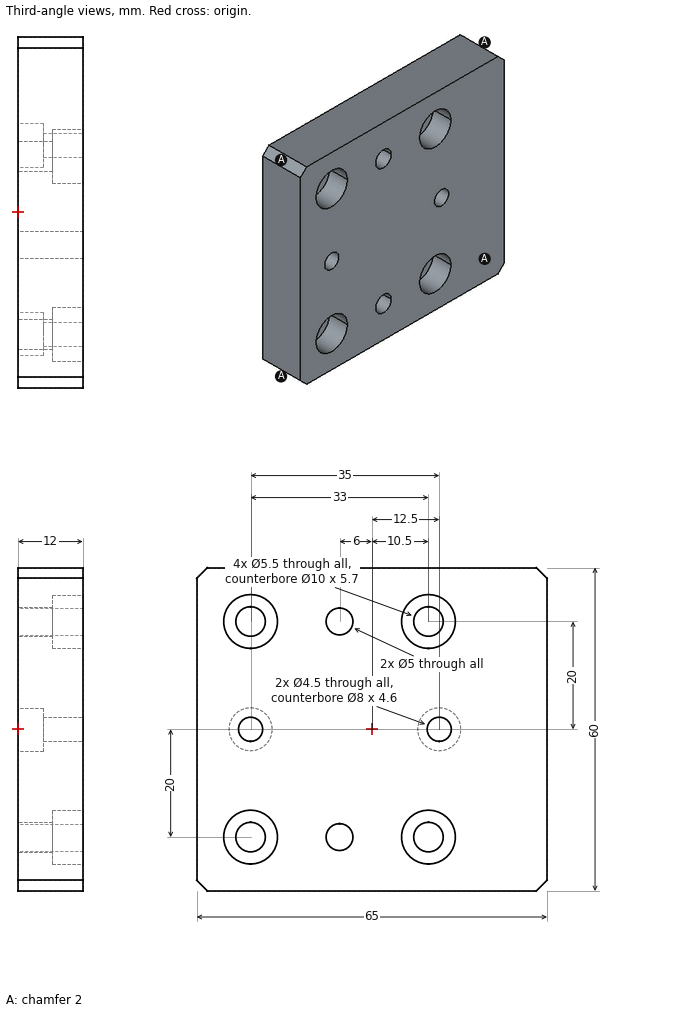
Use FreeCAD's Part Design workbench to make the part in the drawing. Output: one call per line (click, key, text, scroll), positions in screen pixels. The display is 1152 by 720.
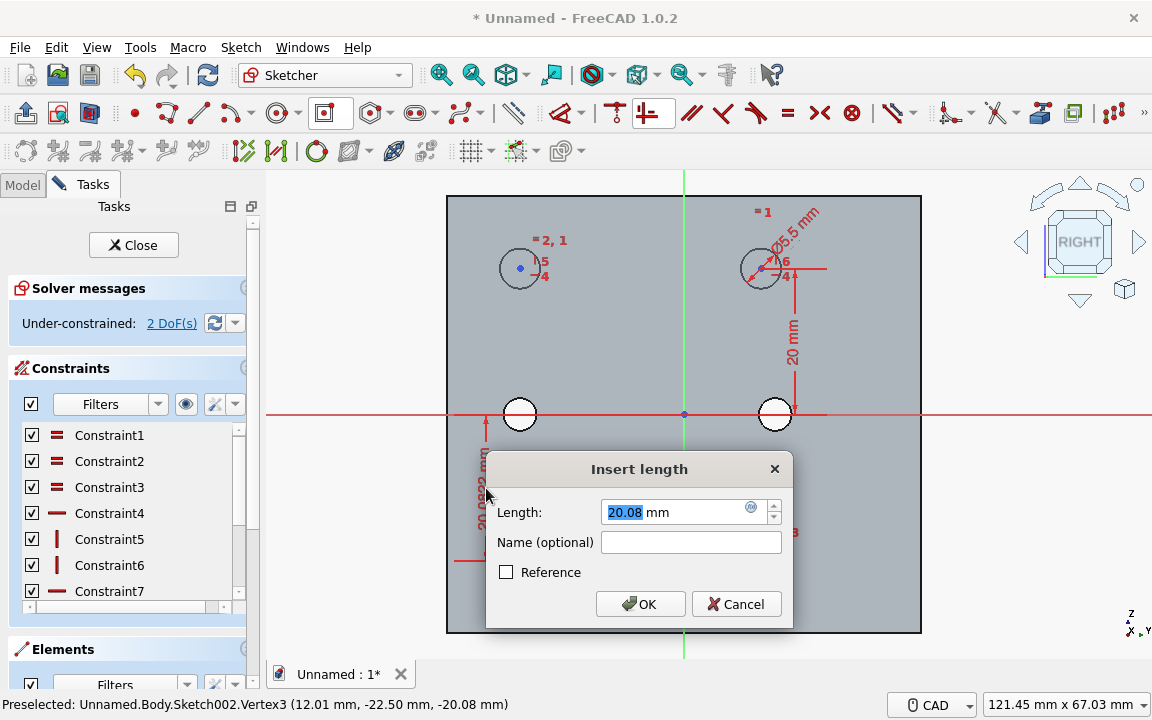
text(20)
key(Return)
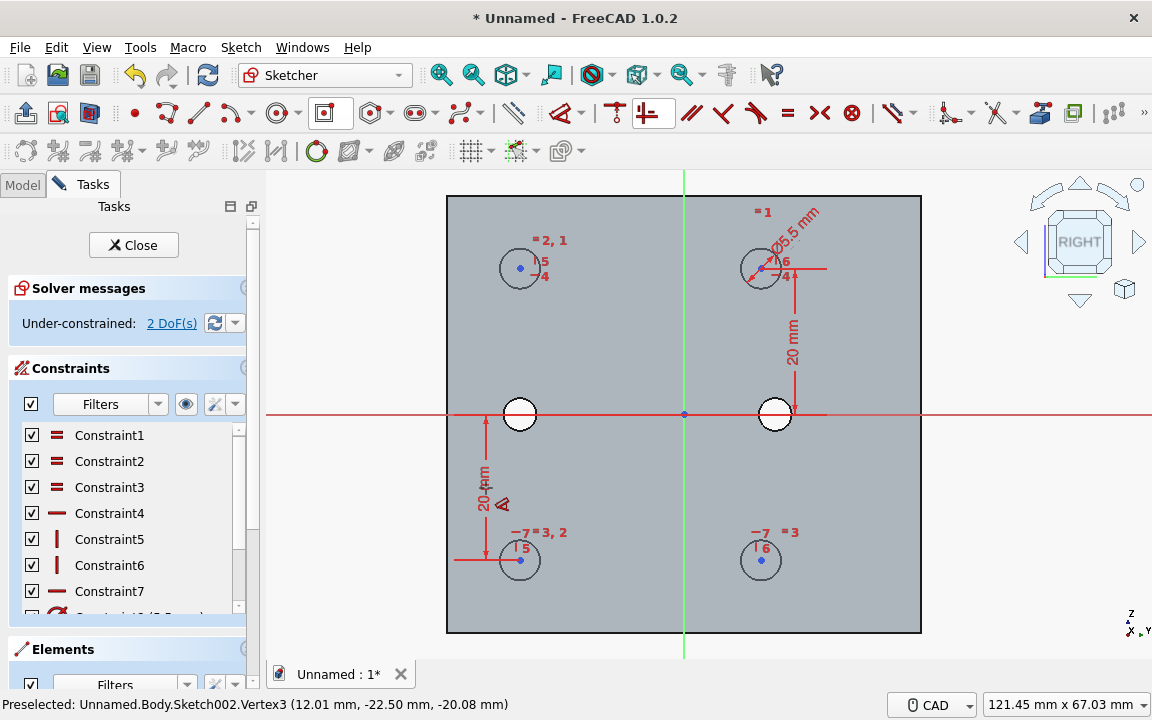
click(761, 269)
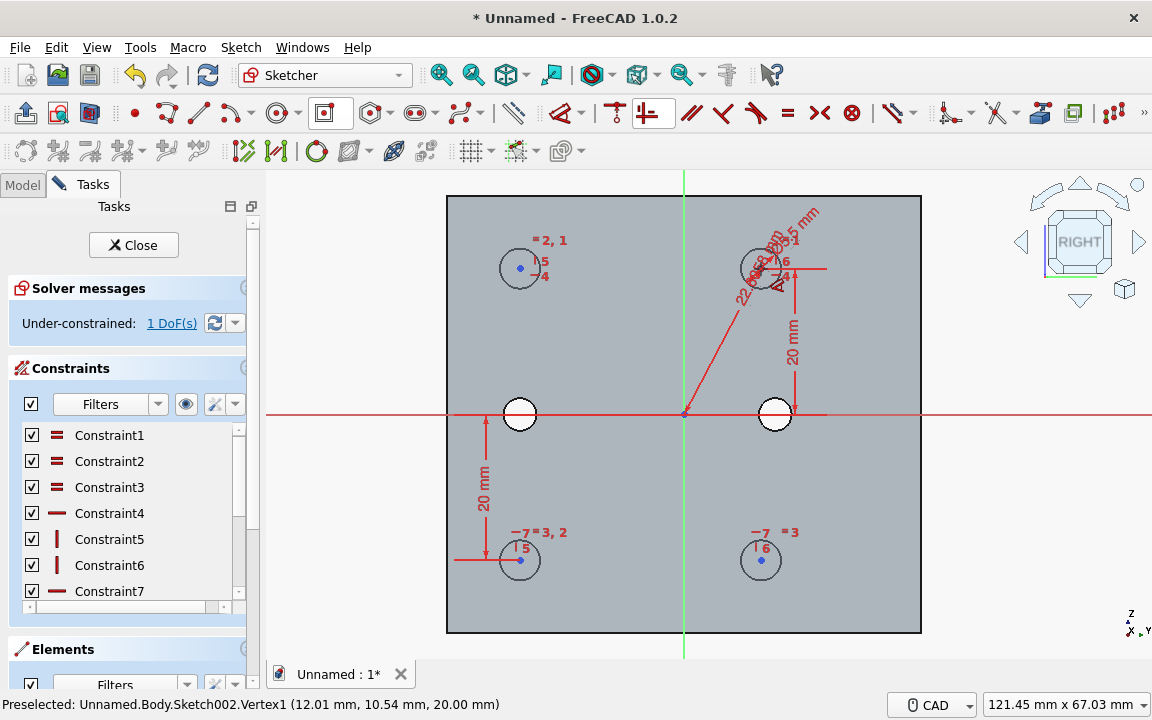
click(520, 269)
click(641, 235)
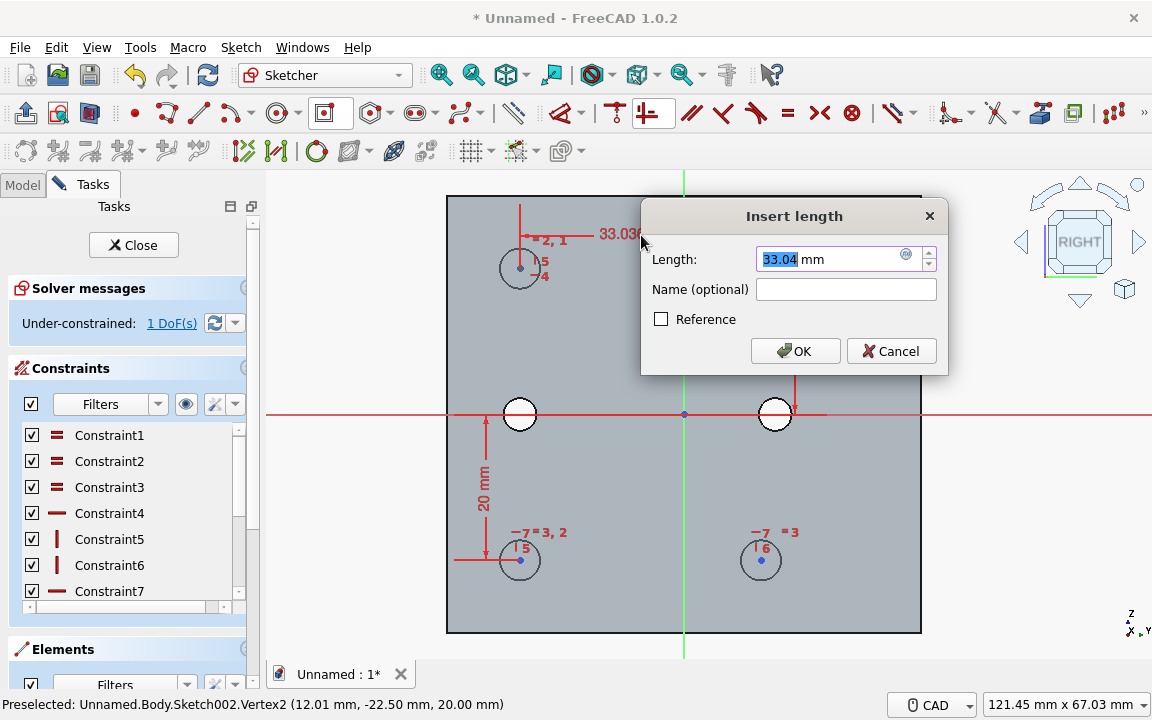
text(33)
key(Return)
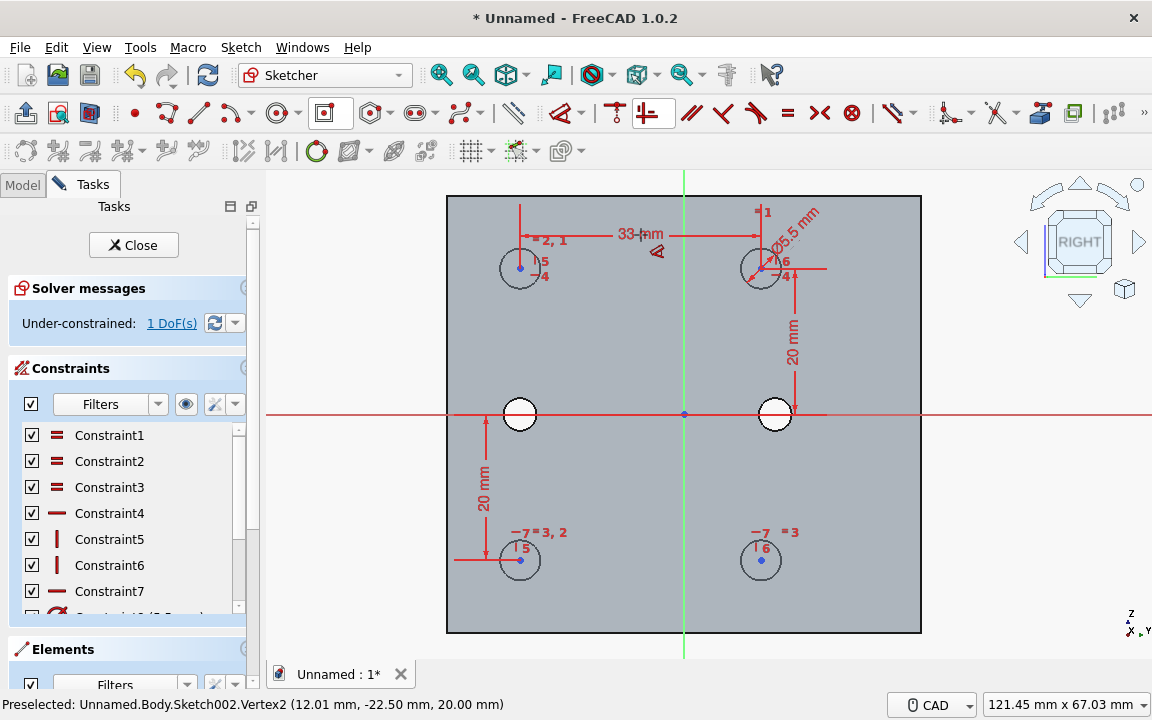
click(761, 269)
click(723, 235)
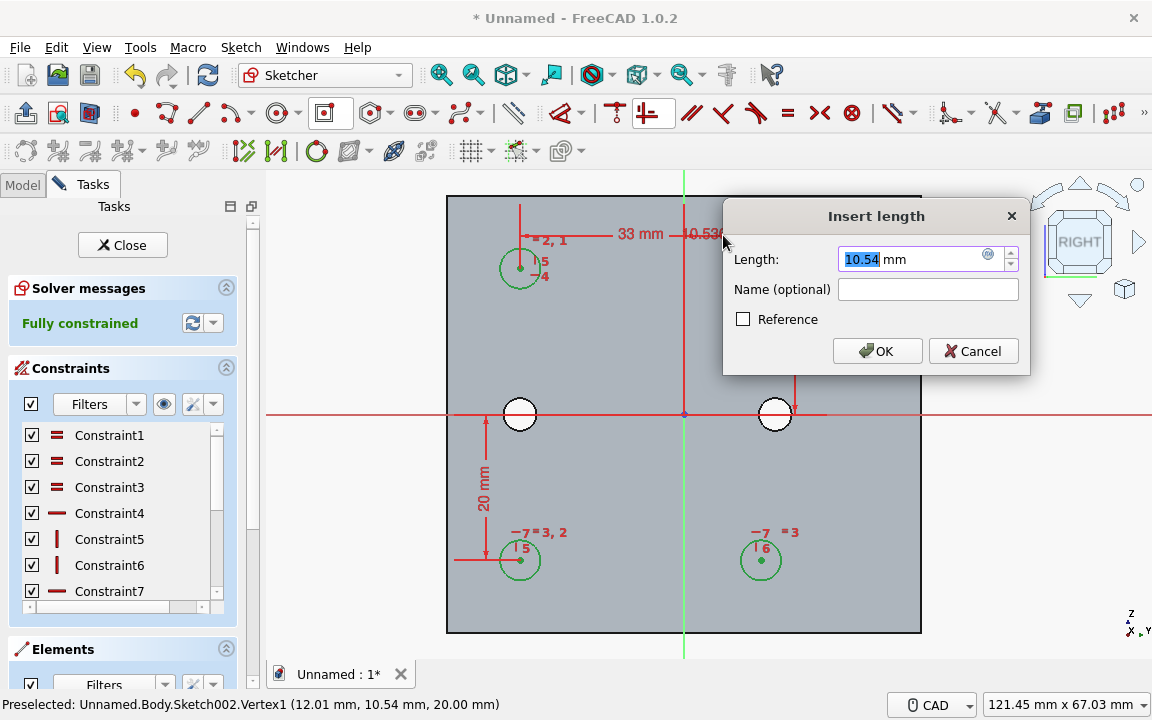
text(10.5)
key(Return)
key(Escape)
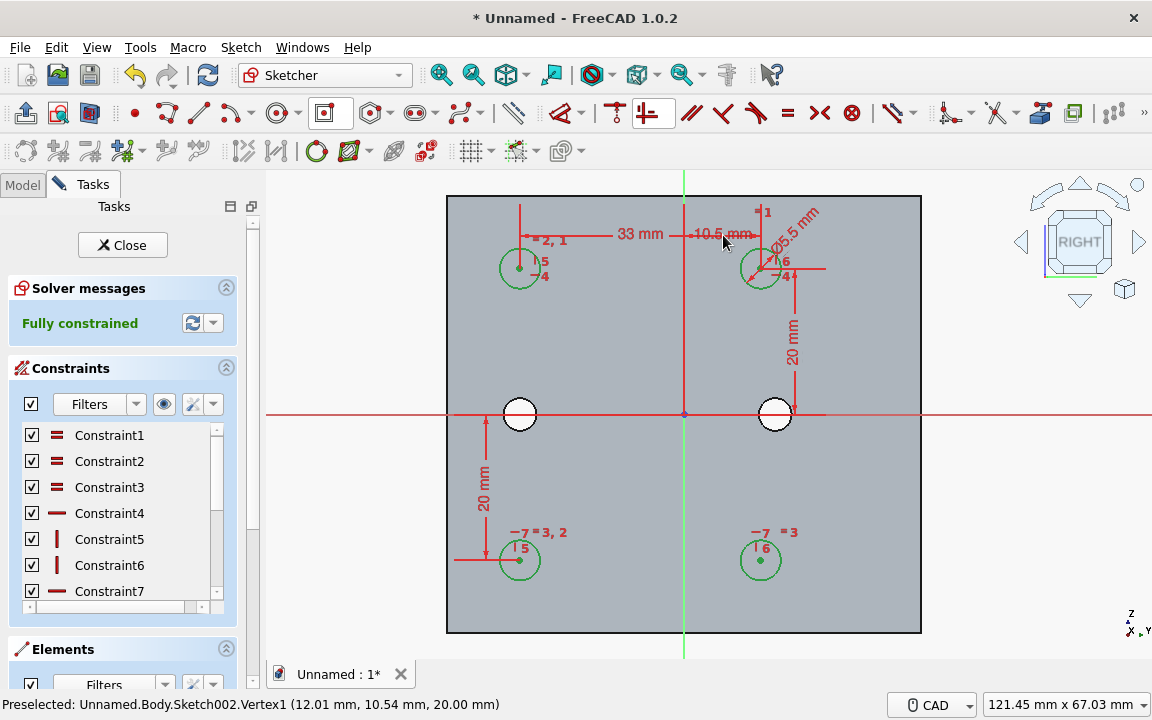
click(123, 245)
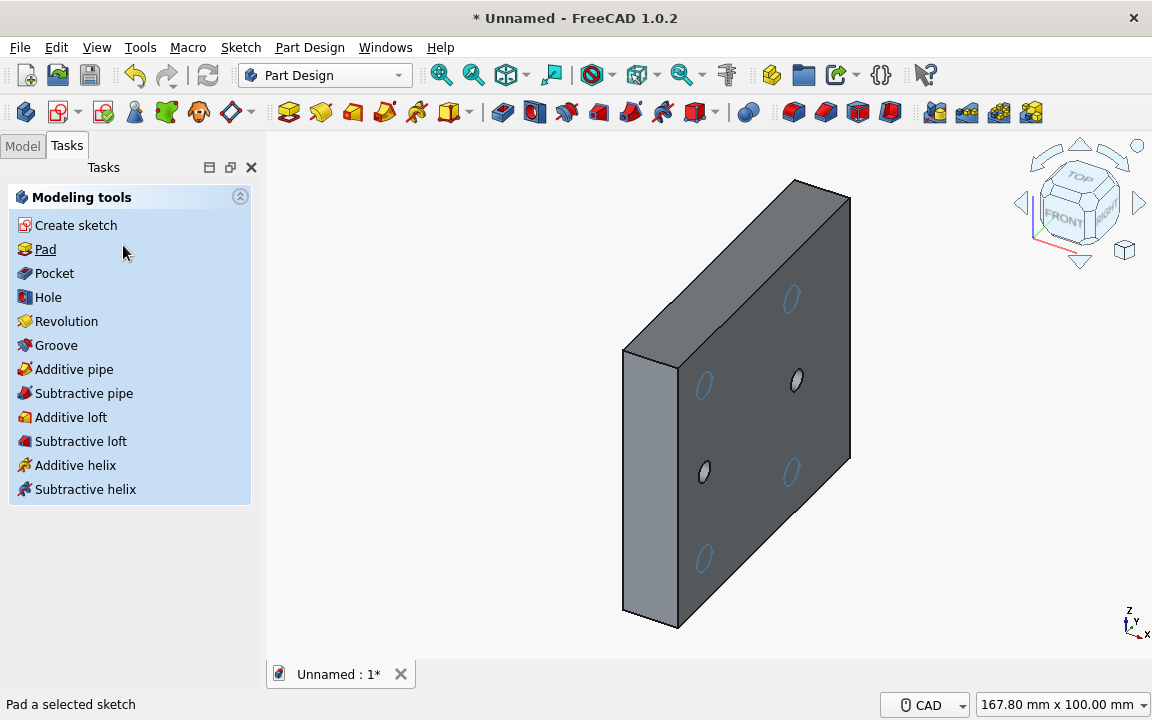
click(536, 112)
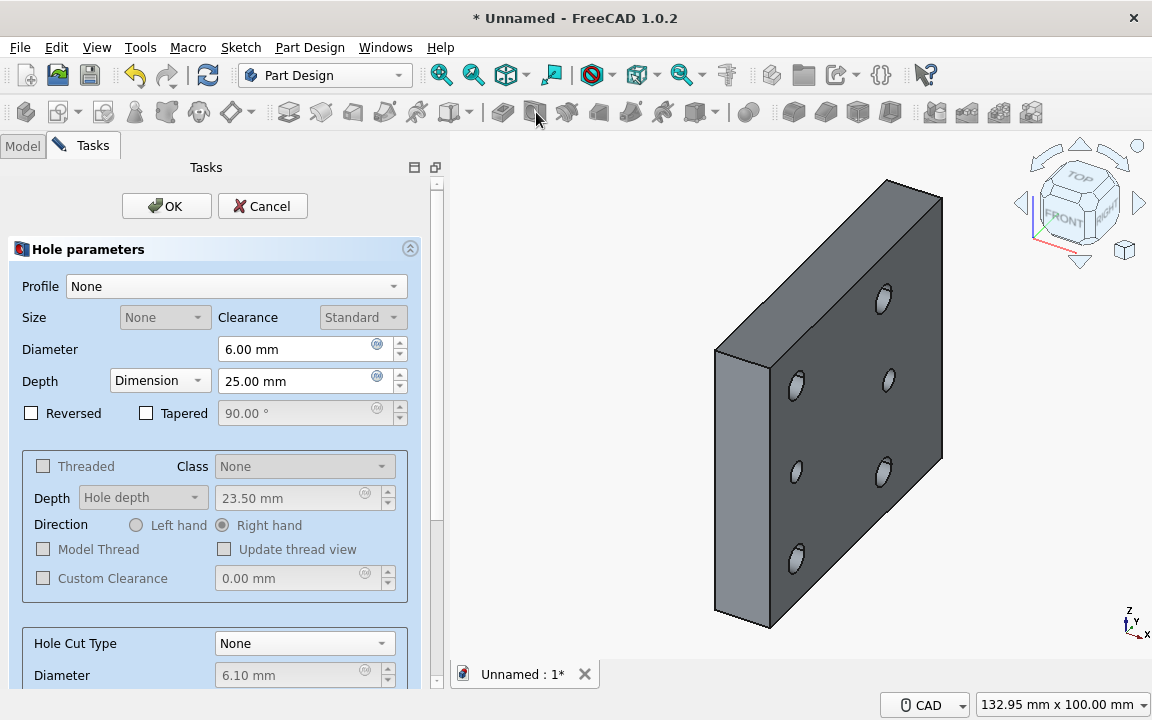
triple_click(305, 349)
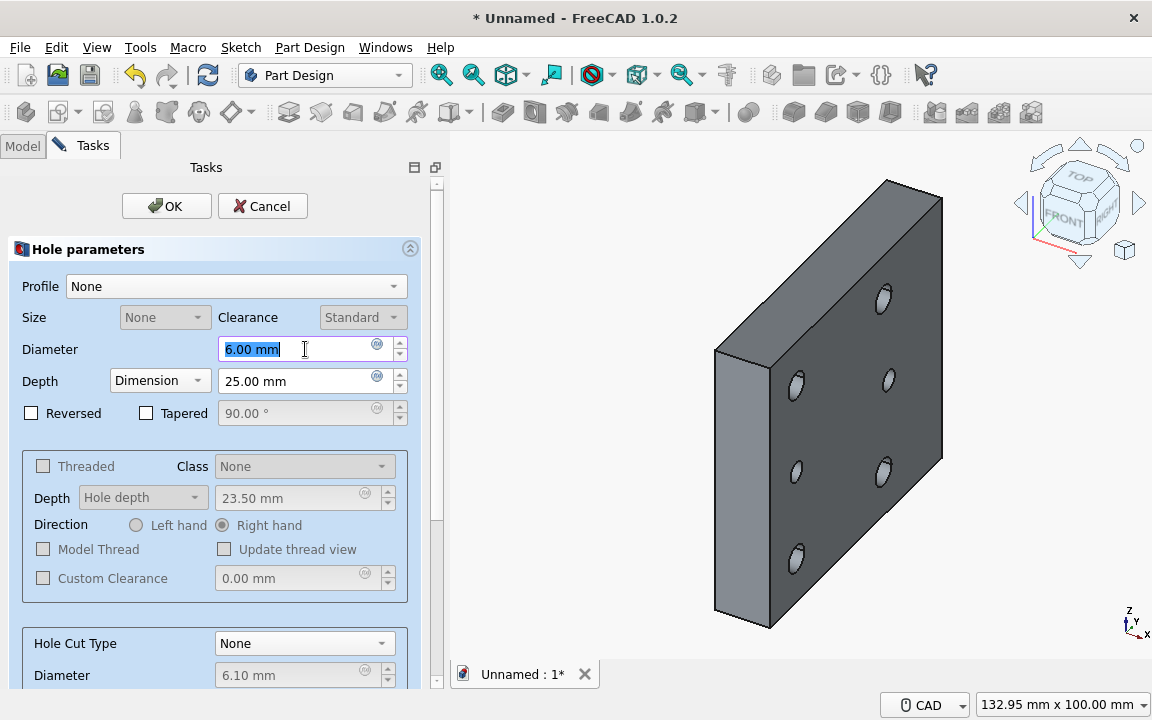
text(5.5)
key(Tab)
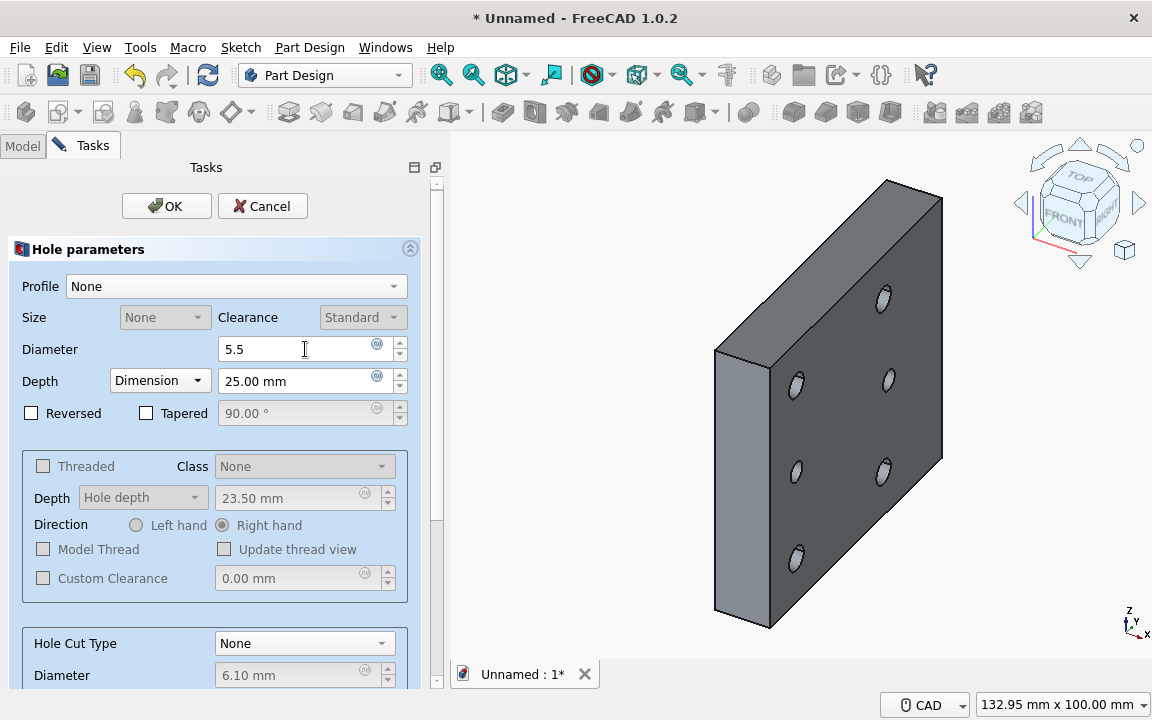
click(161, 380)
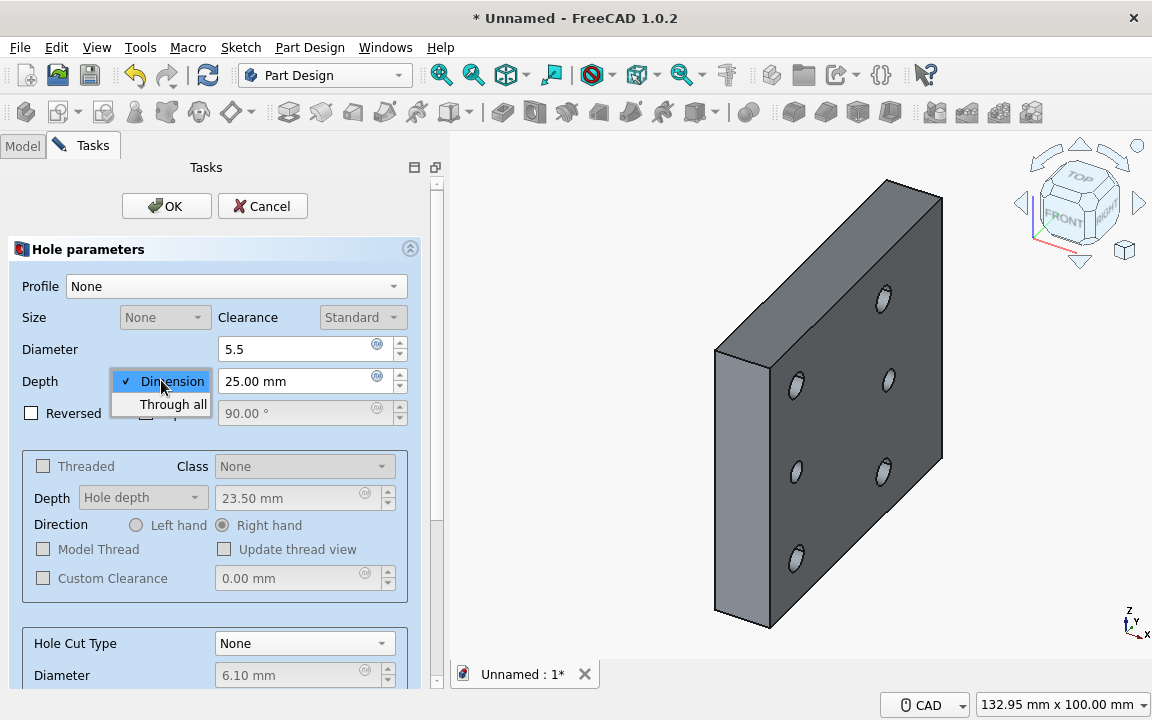
click(160, 404)